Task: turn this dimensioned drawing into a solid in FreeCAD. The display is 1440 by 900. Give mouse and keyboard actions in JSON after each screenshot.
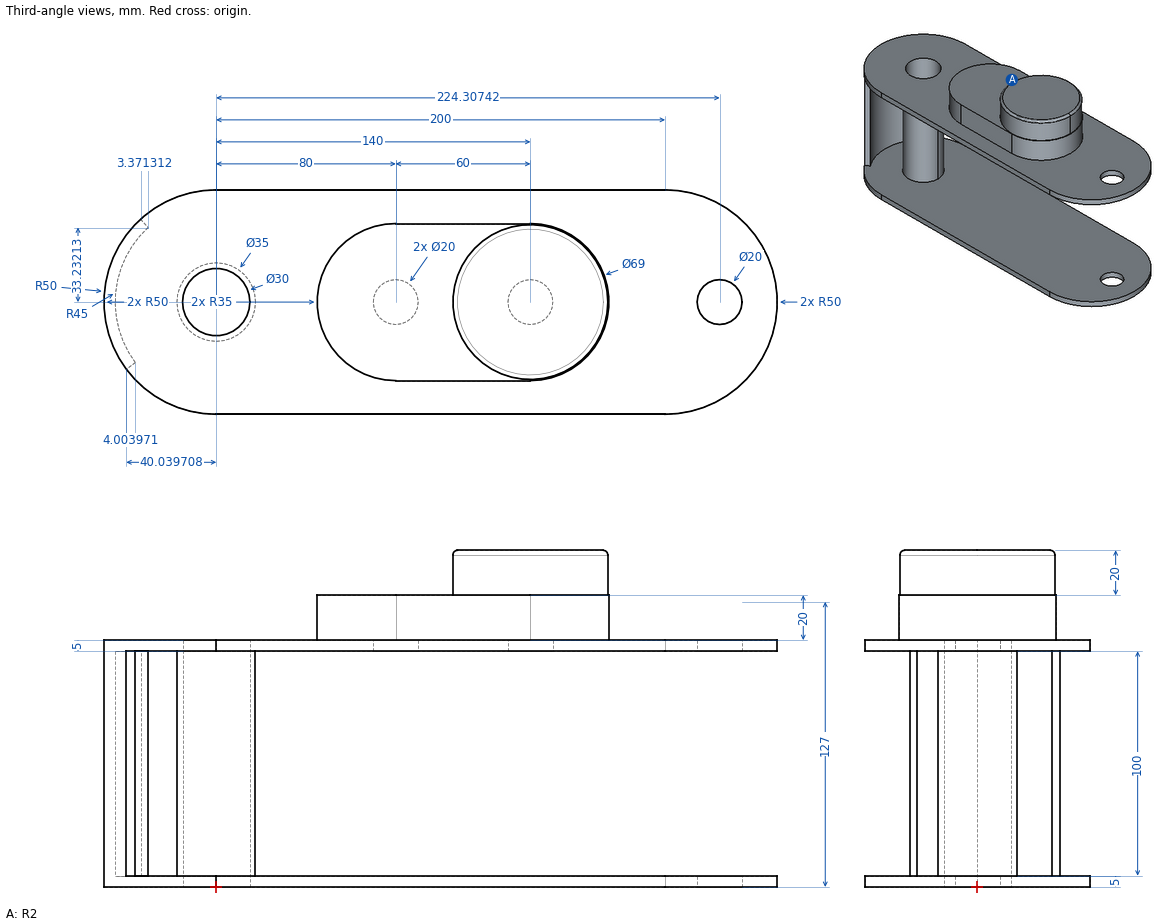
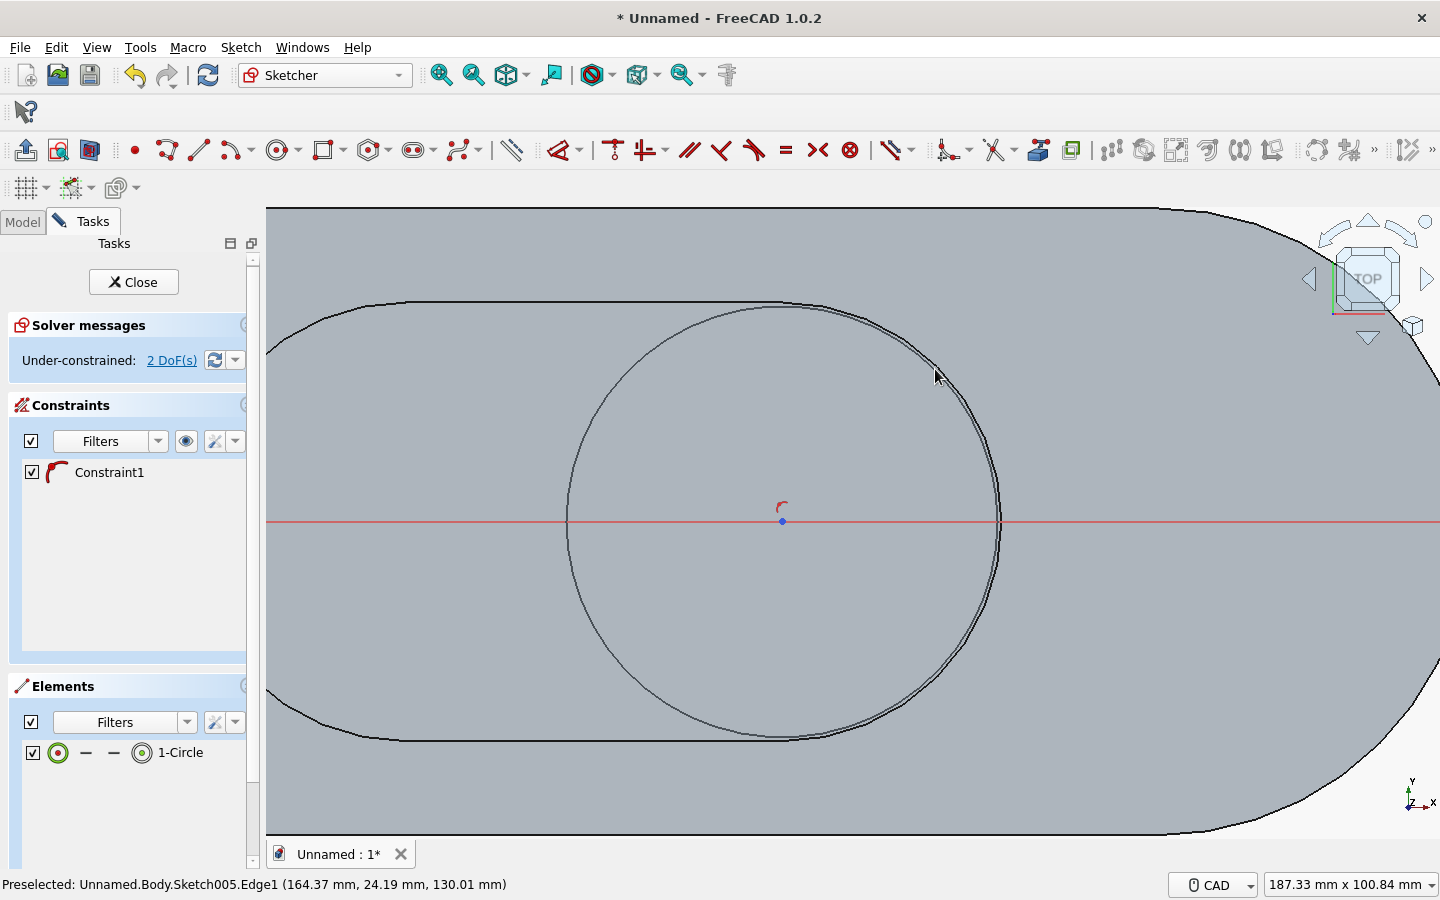
{"action": "left_click", "coordinate": [558, 150]}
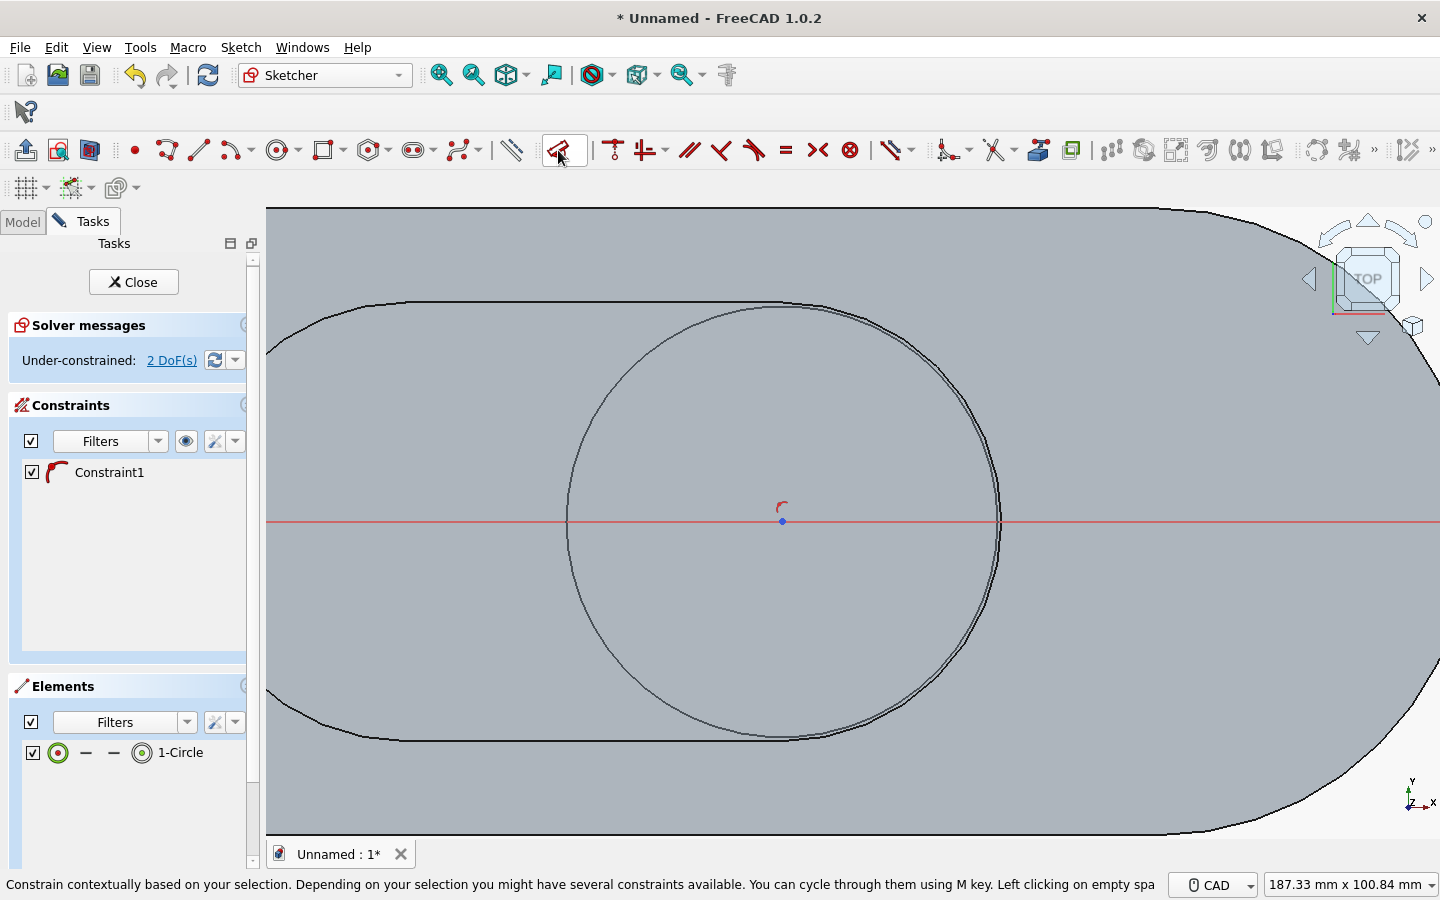
{"action": "left_click", "coordinate": [934, 369]}
{"action": "left_click", "coordinate": [957, 346]}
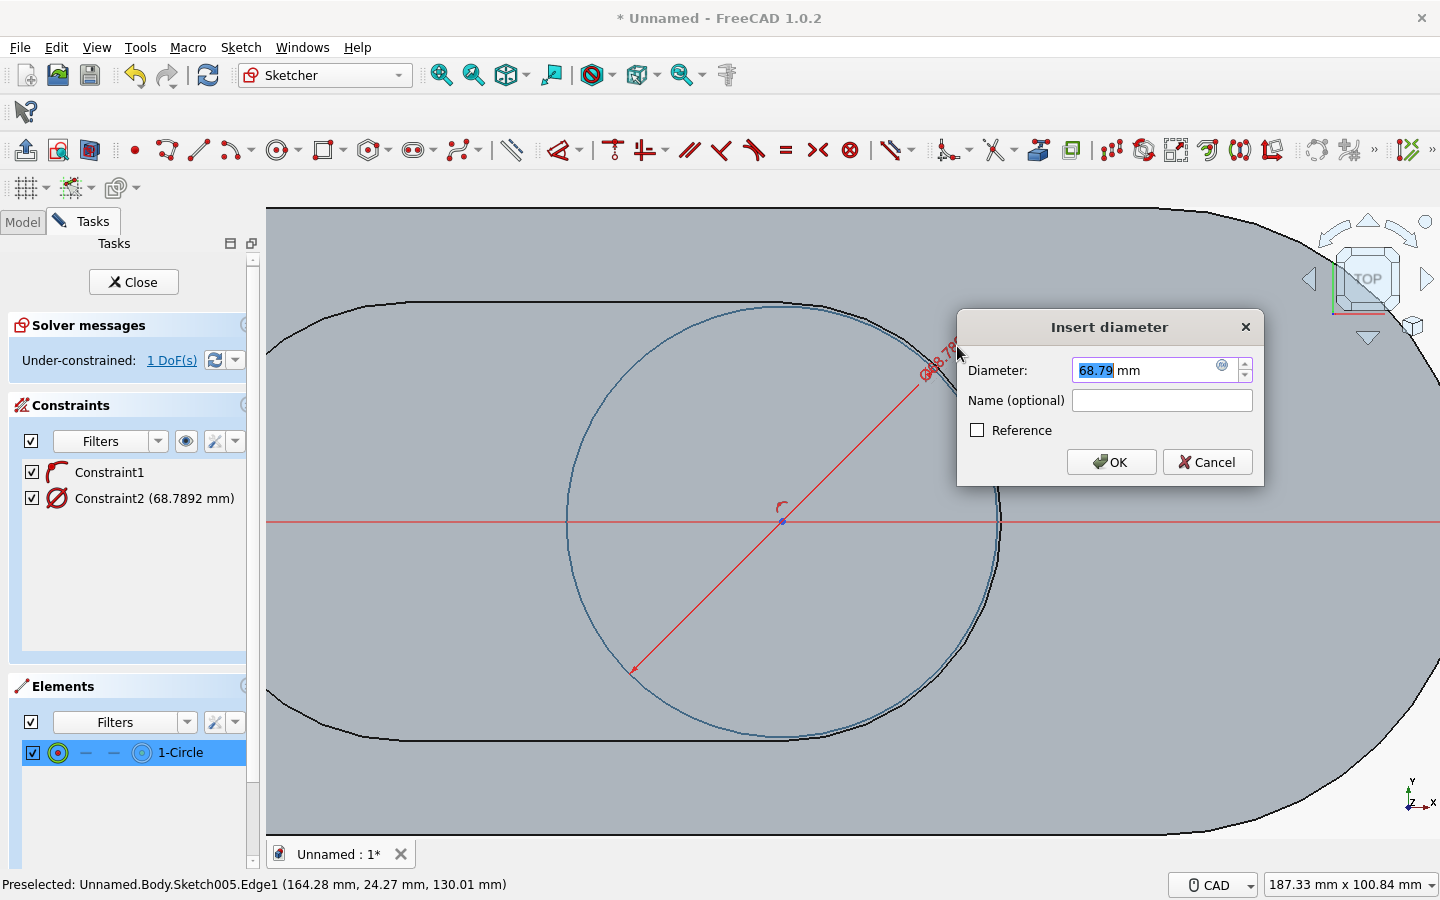
{"action": "type", "text": "69"}
{"action": "key", "text": "Return"}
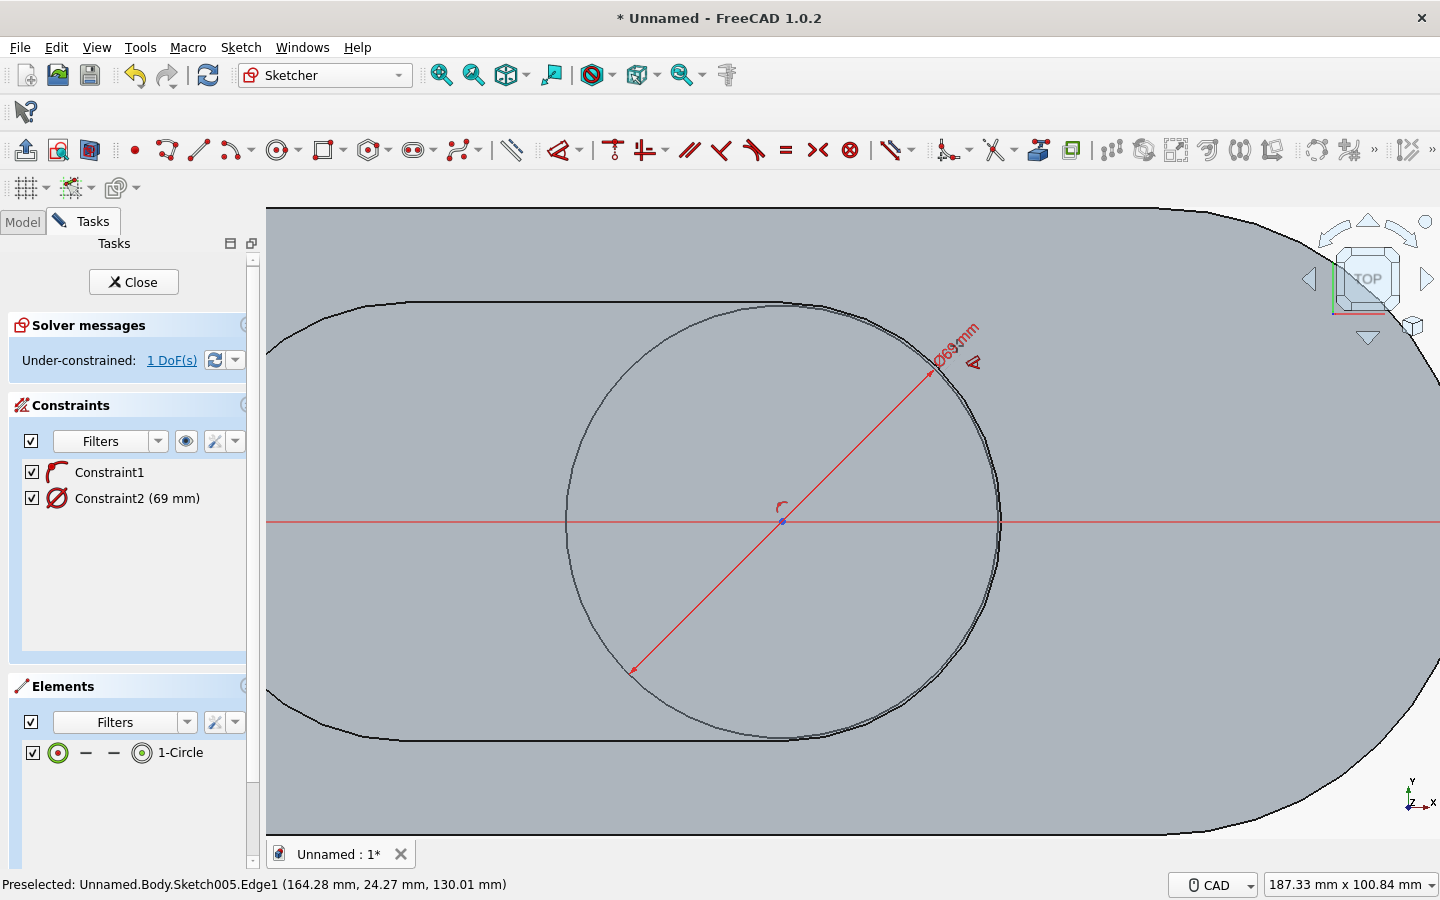
{"action": "left_click", "coordinate": [782, 522]}
{"action": "left_click", "coordinate": [538, 556]}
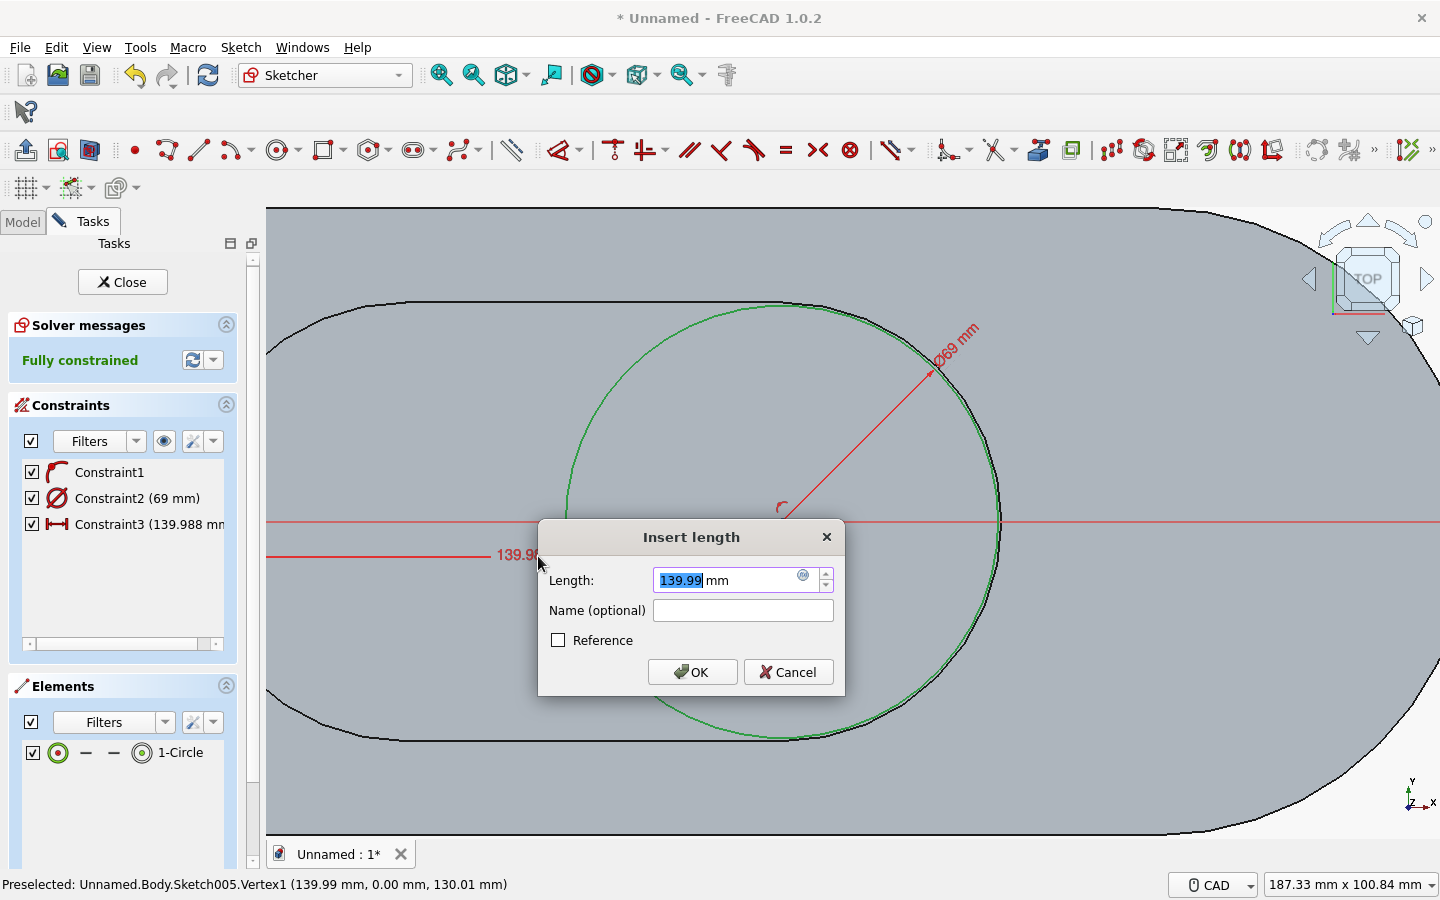
{"action": "type", "text": "140"}
{"action": "key", "text": "Return"}
{"action": "key", "text": "Escape"}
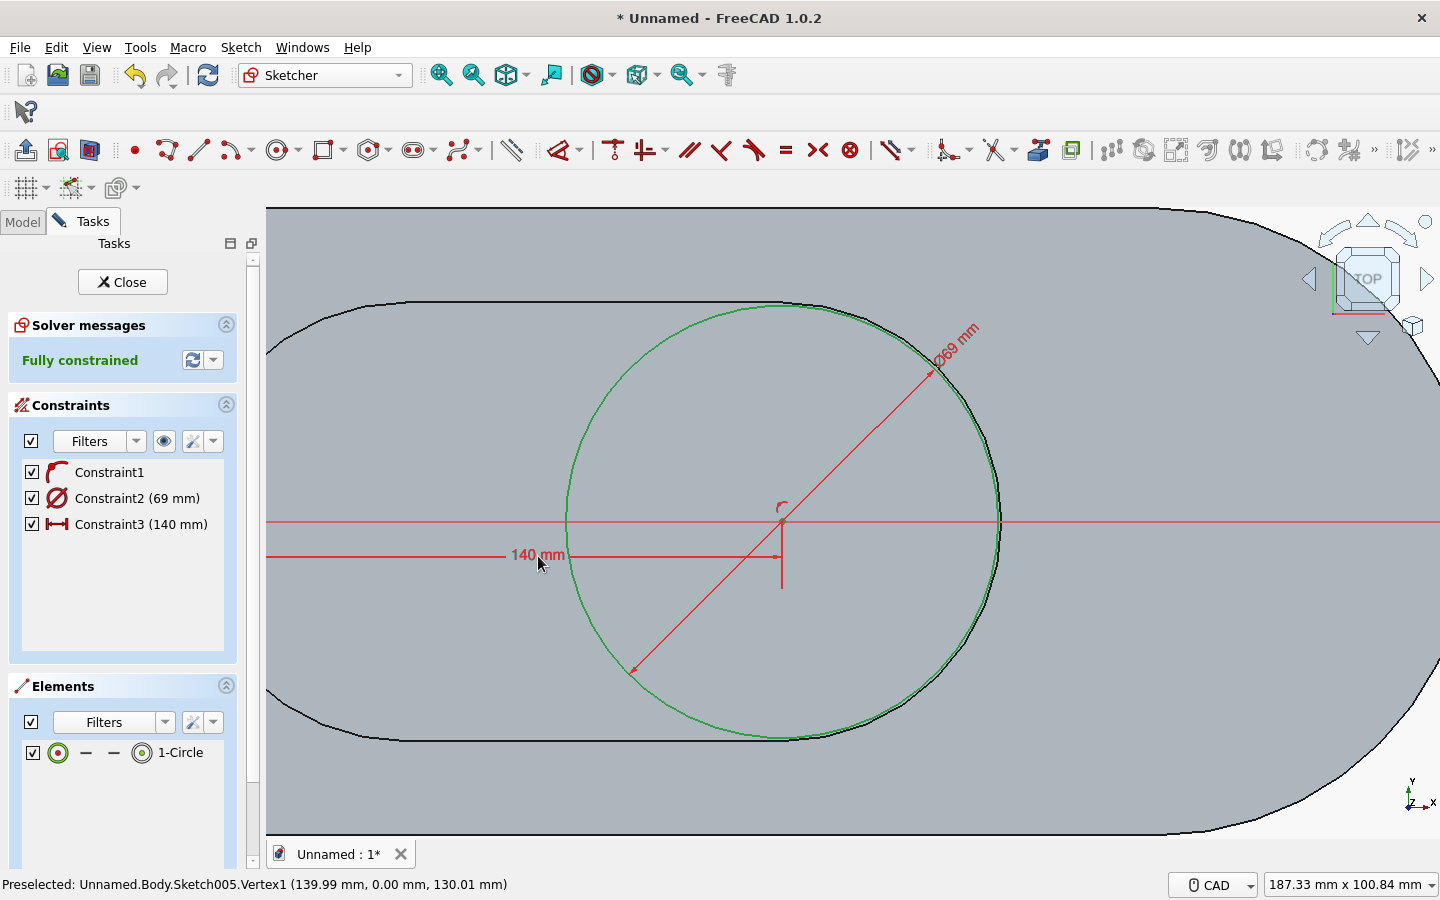
{"action": "left_click", "coordinate": [123, 282]}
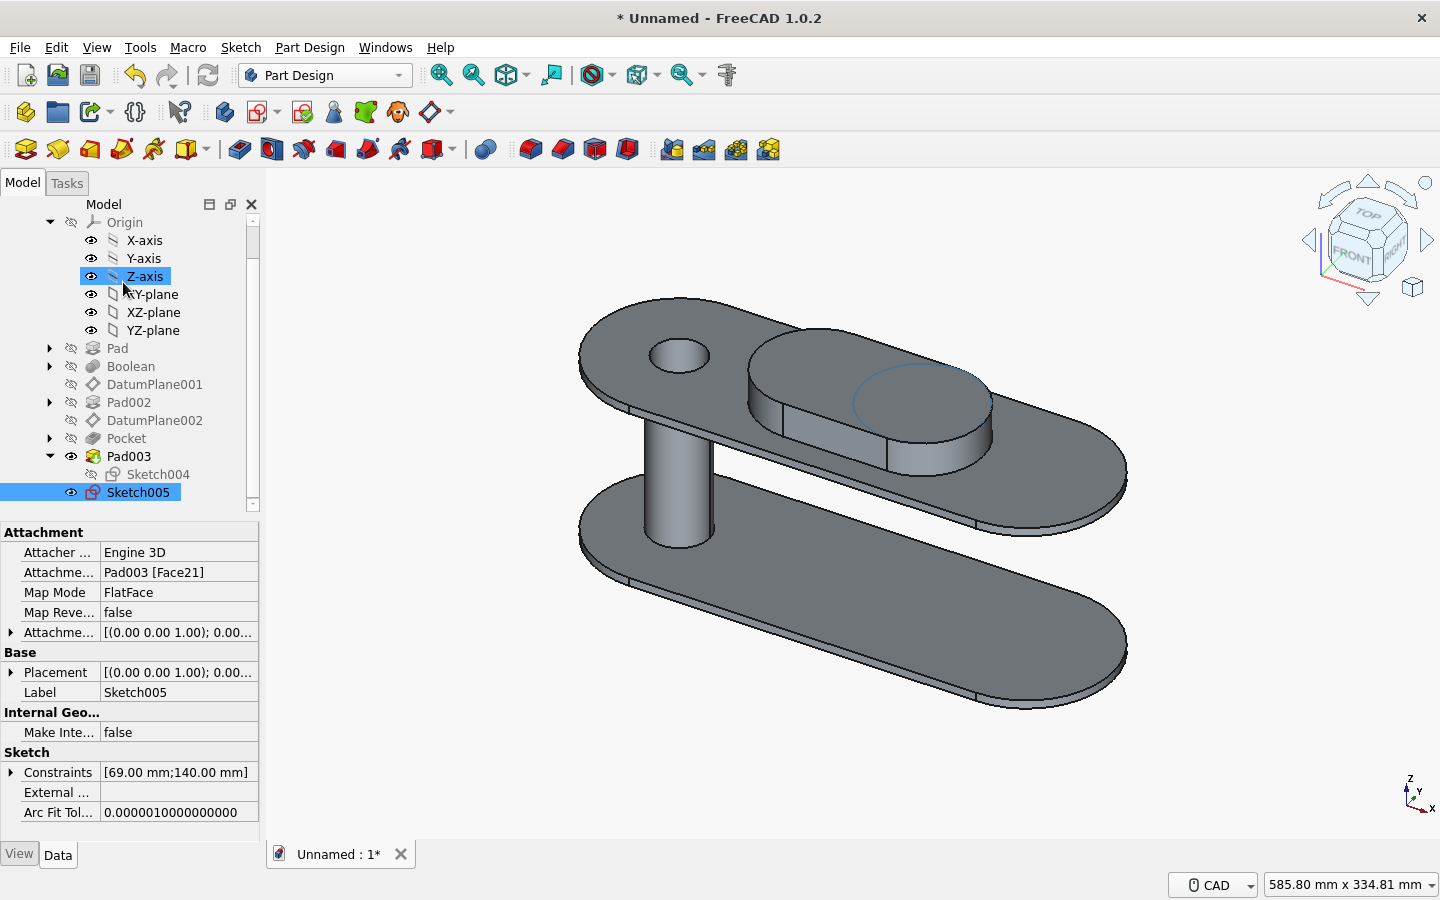
{"action": "left_click", "coordinate": [26, 150]}